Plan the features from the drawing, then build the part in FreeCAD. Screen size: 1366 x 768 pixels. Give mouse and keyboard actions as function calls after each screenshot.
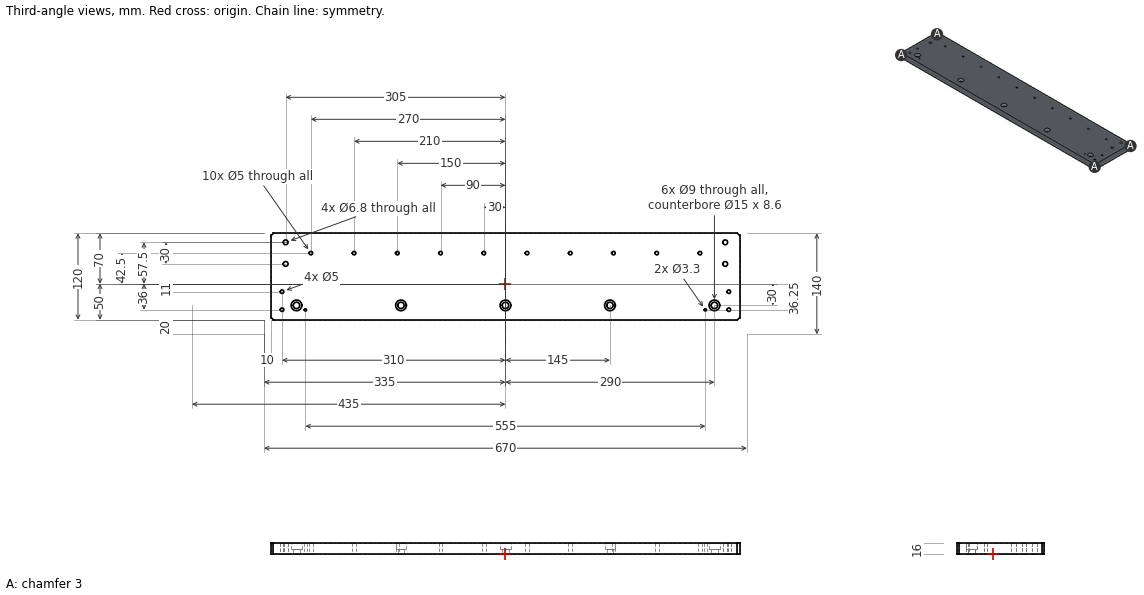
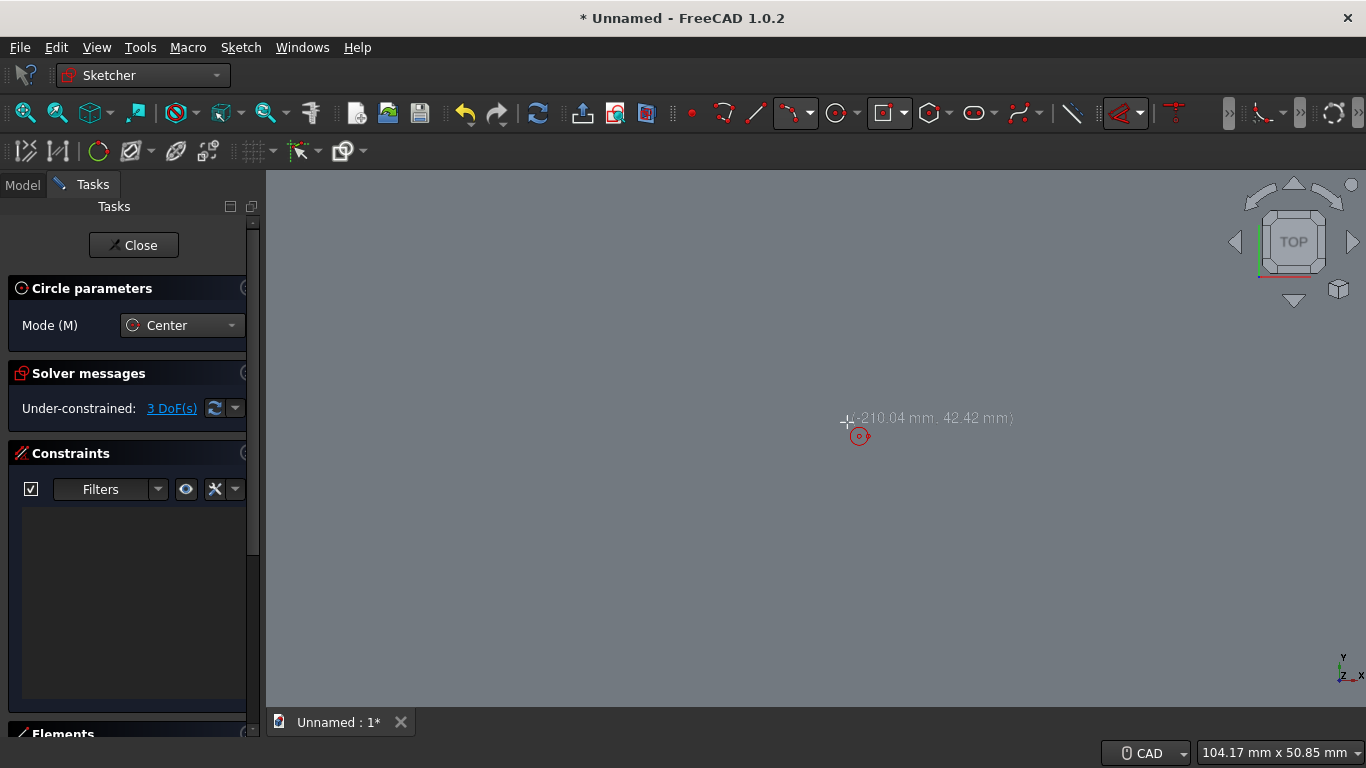
scroll(459, 414, down, 11)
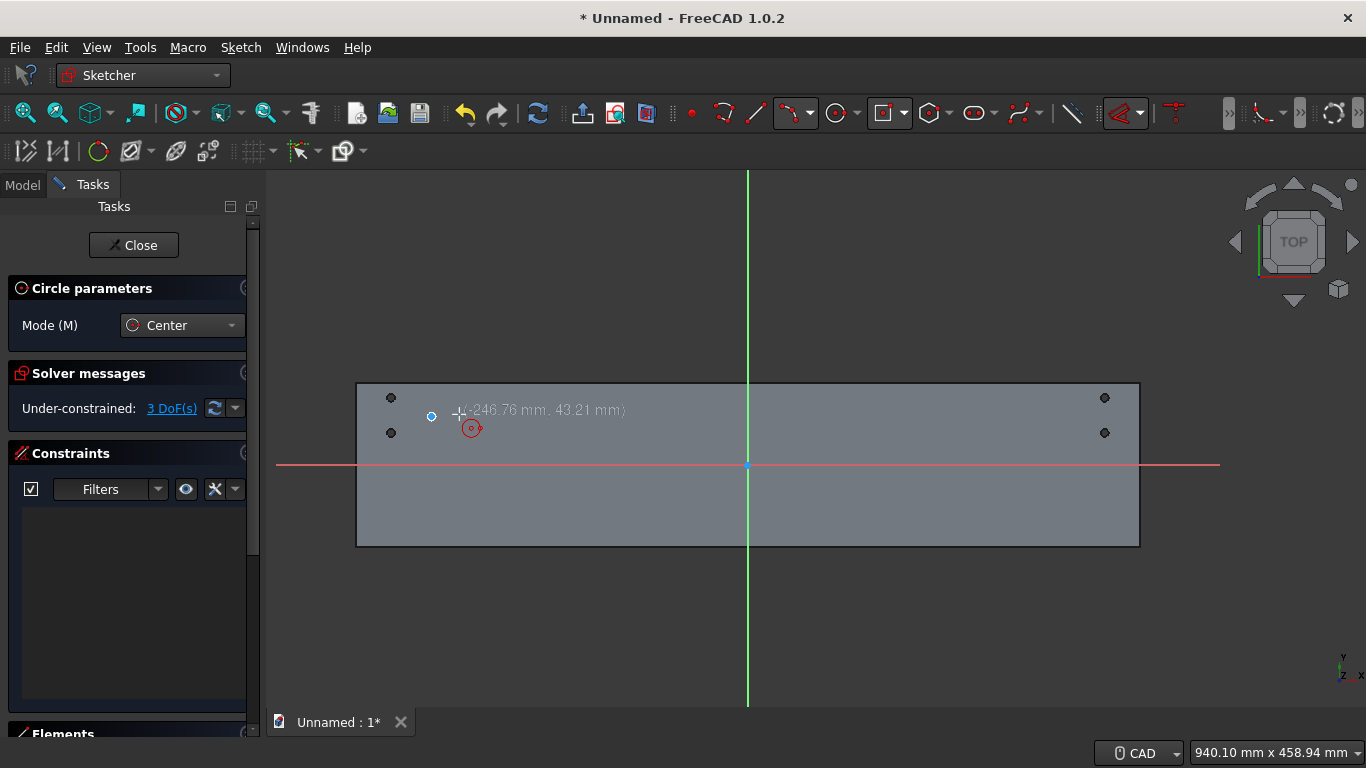
click(502, 415)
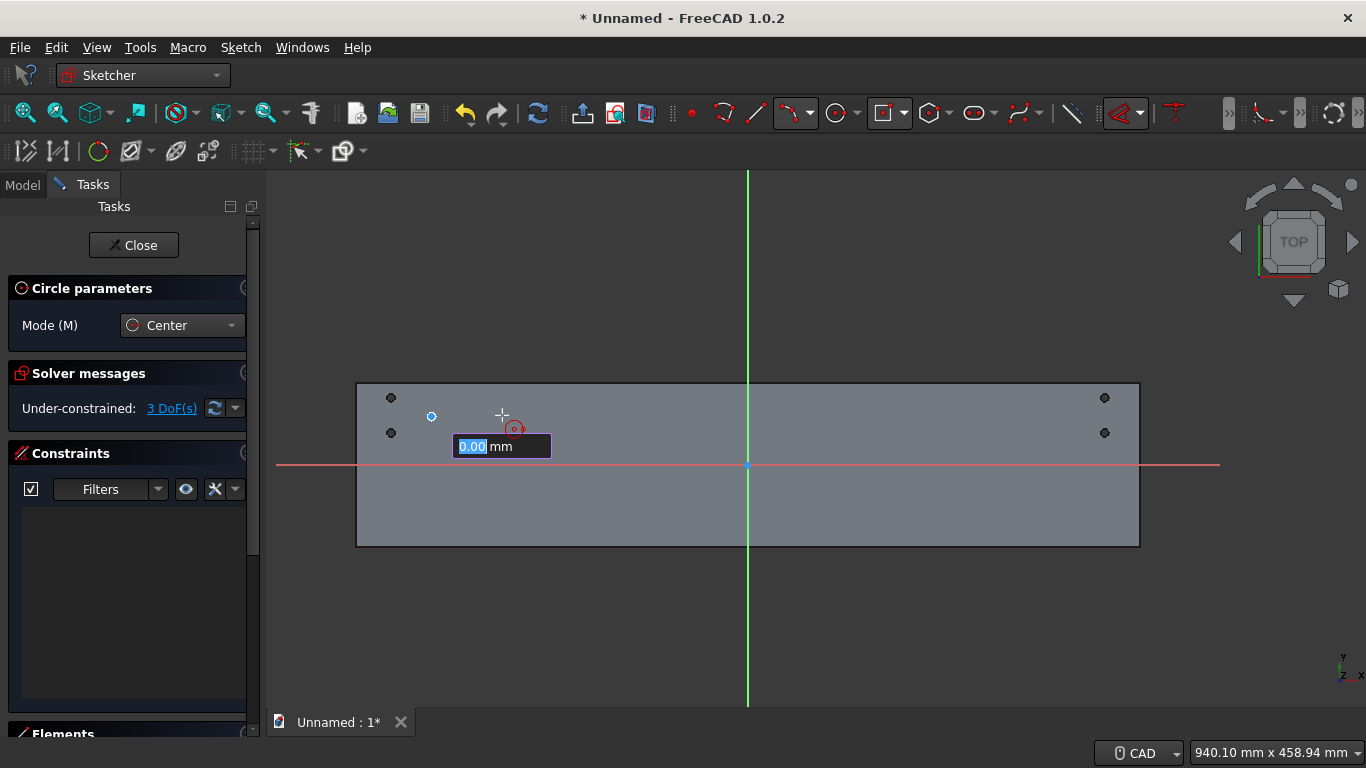
scroll(504, 413, up, 9)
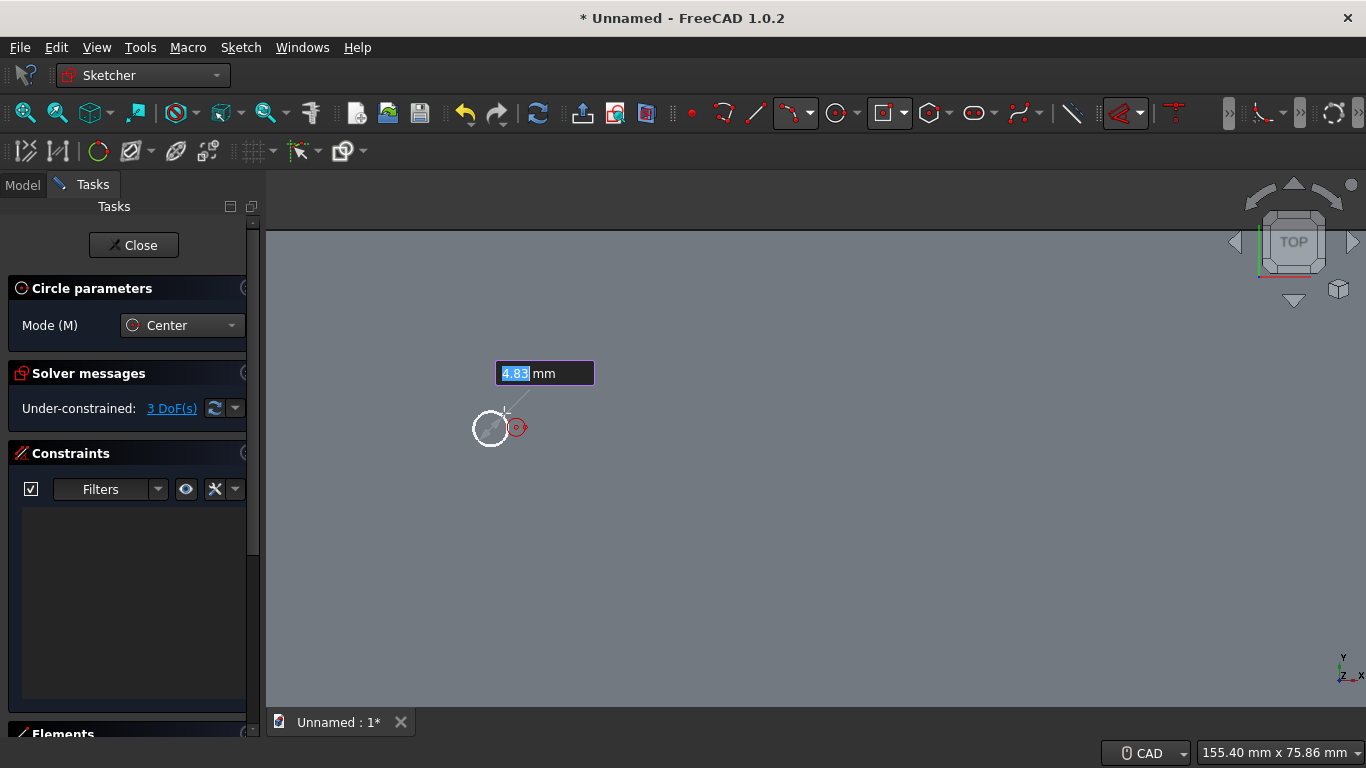
click(504, 412)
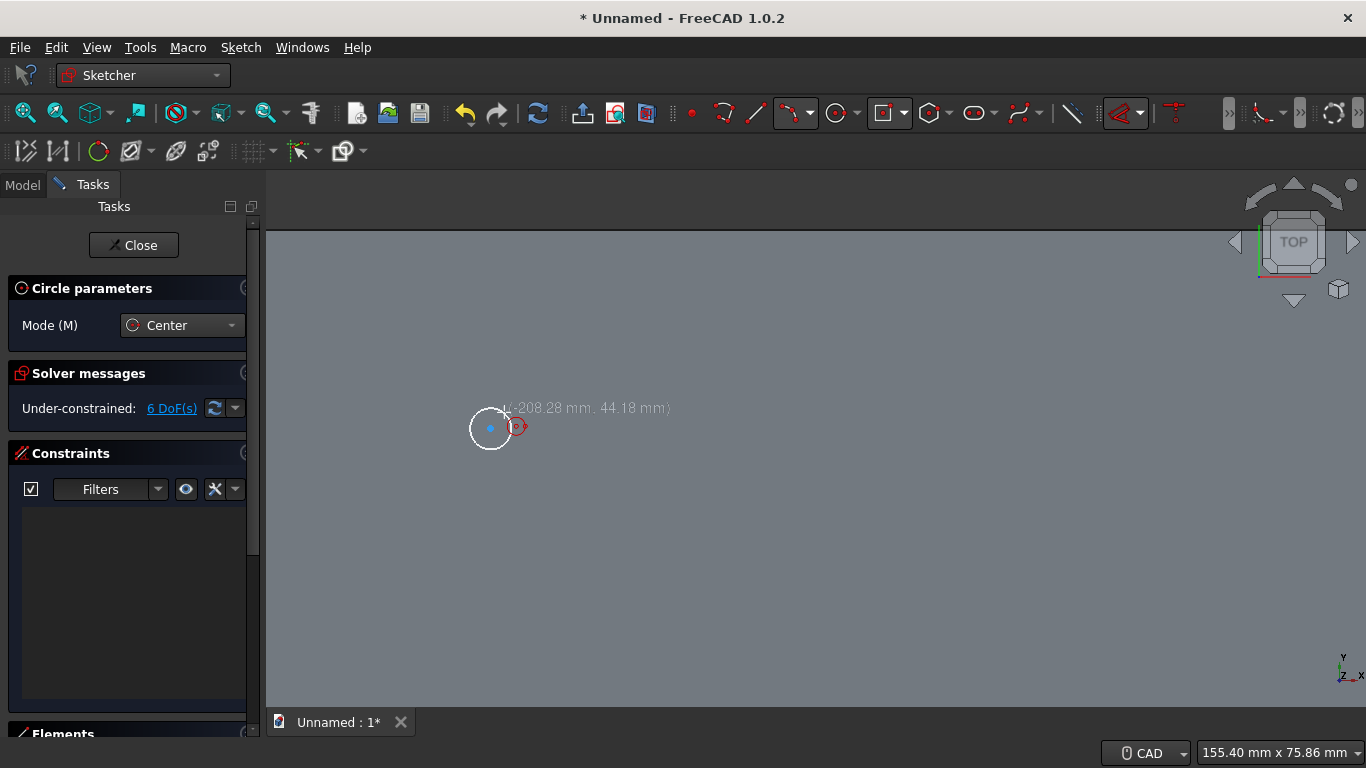
scroll(917, 425, up, 2)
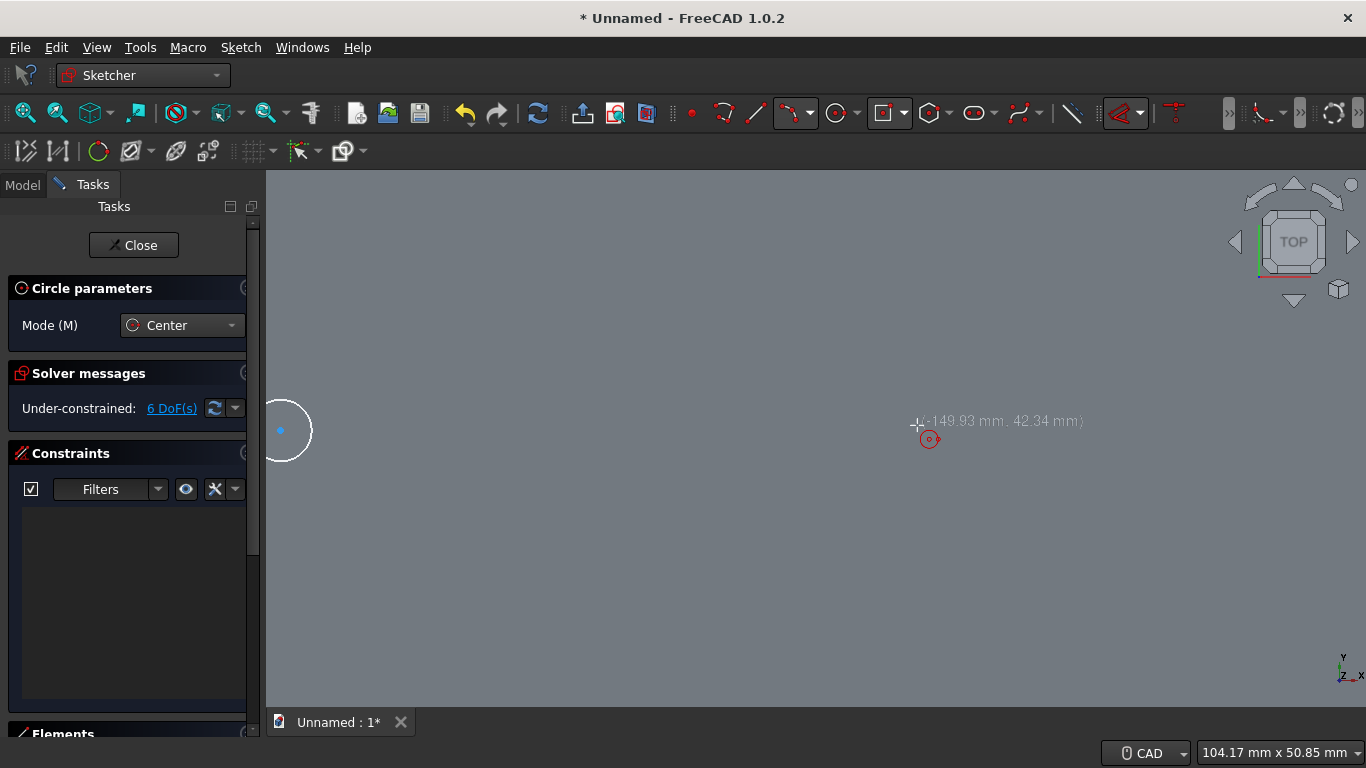
scroll(529, 414, down, 11)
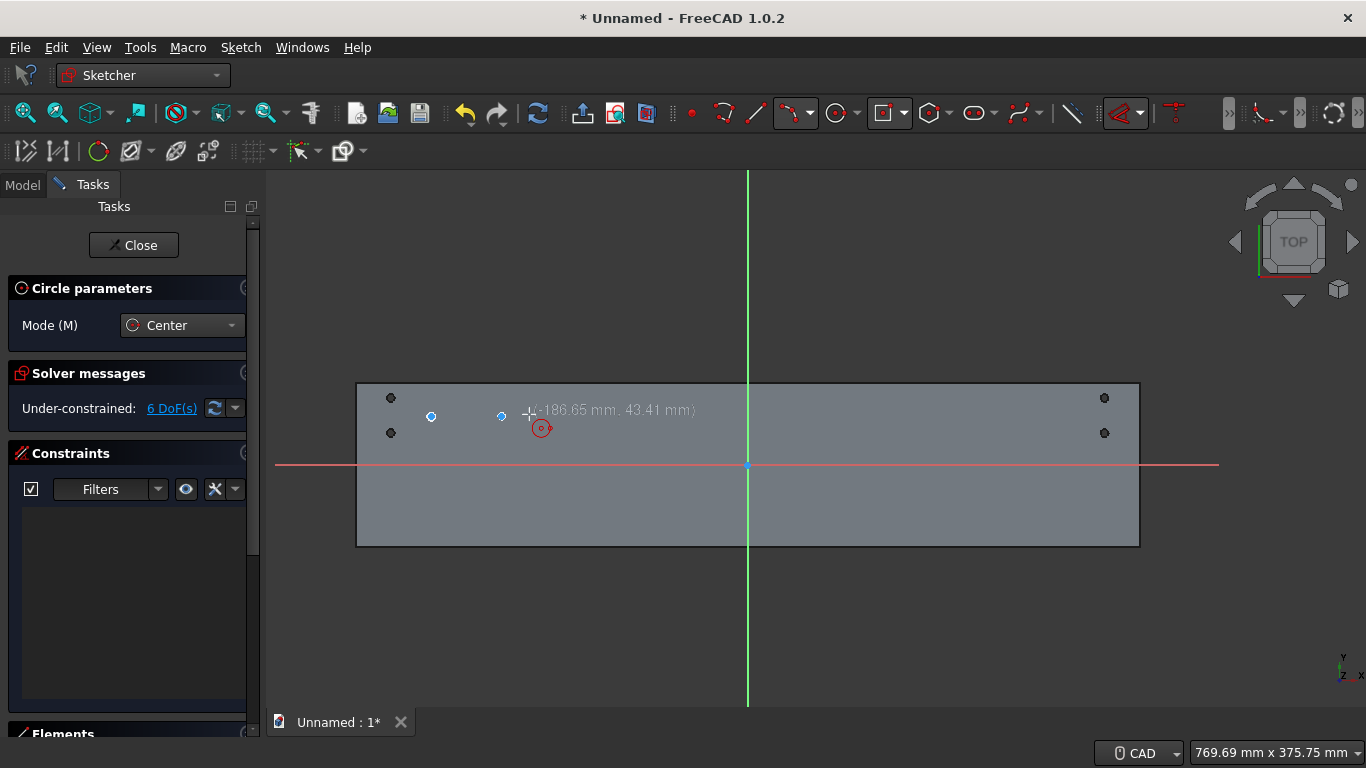
click(572, 416)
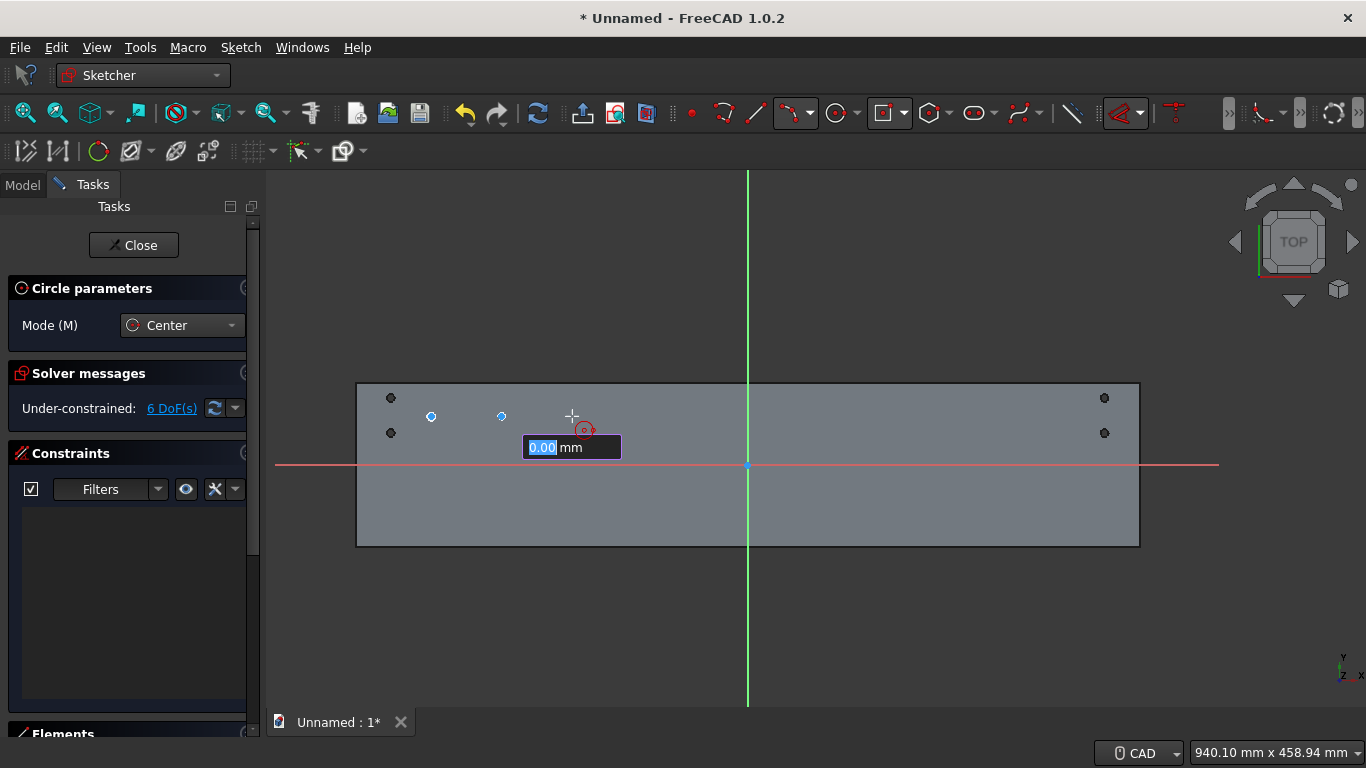
scroll(574, 414, up, 9)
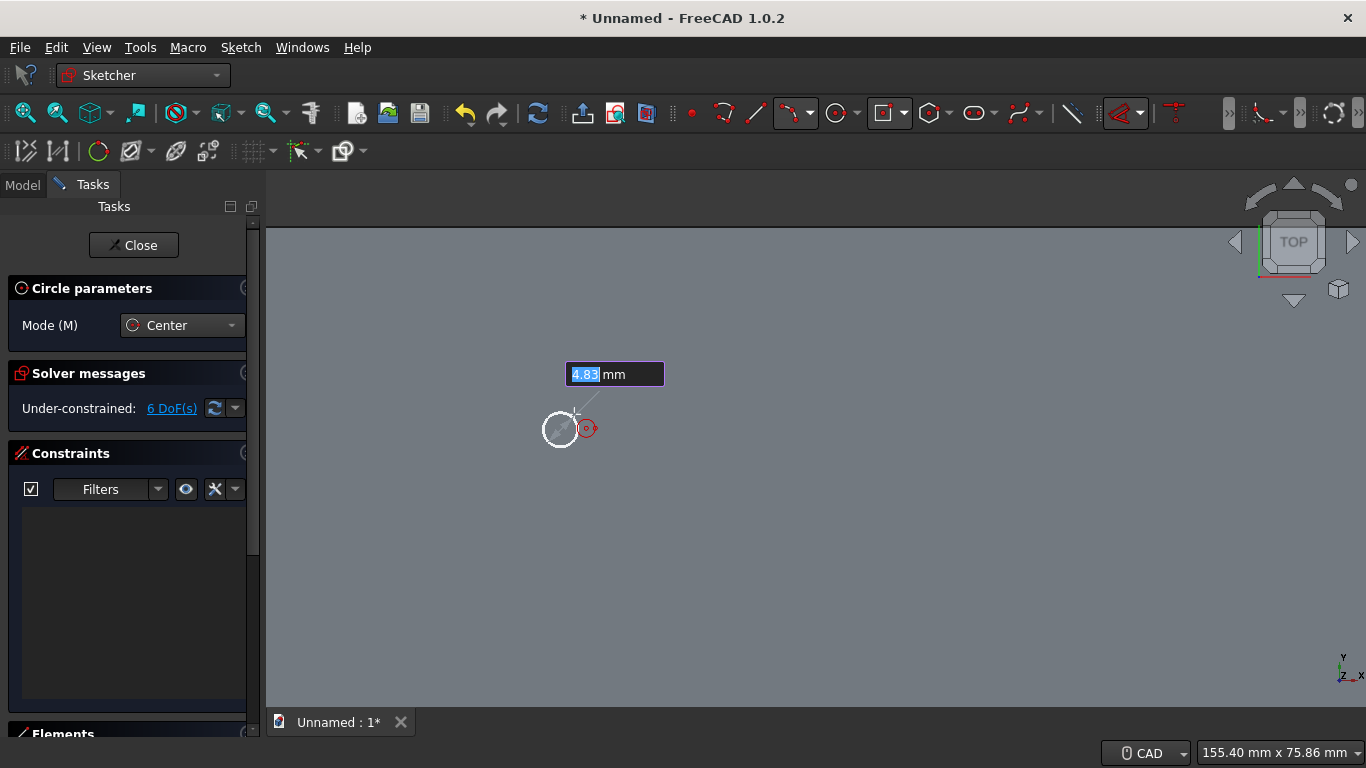
click(574, 409)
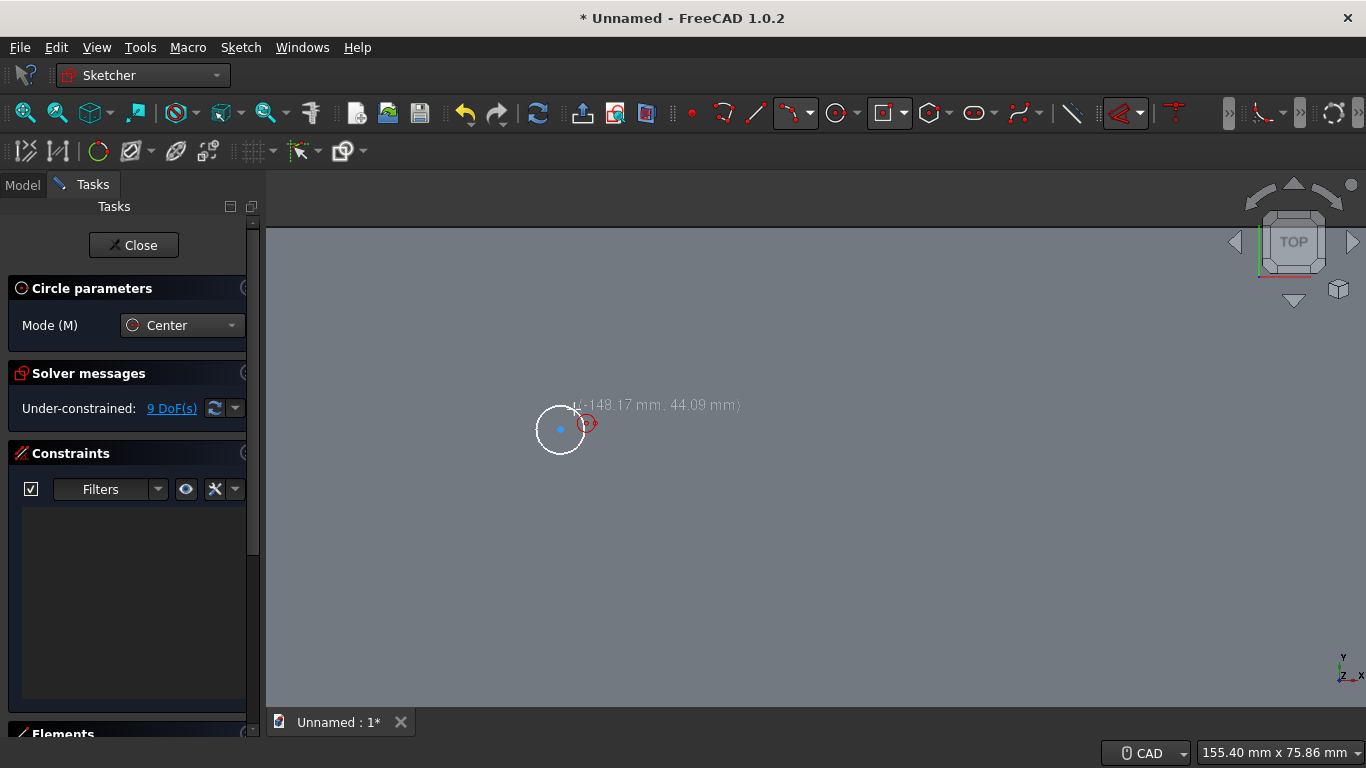
scroll(986, 421, up, 2)